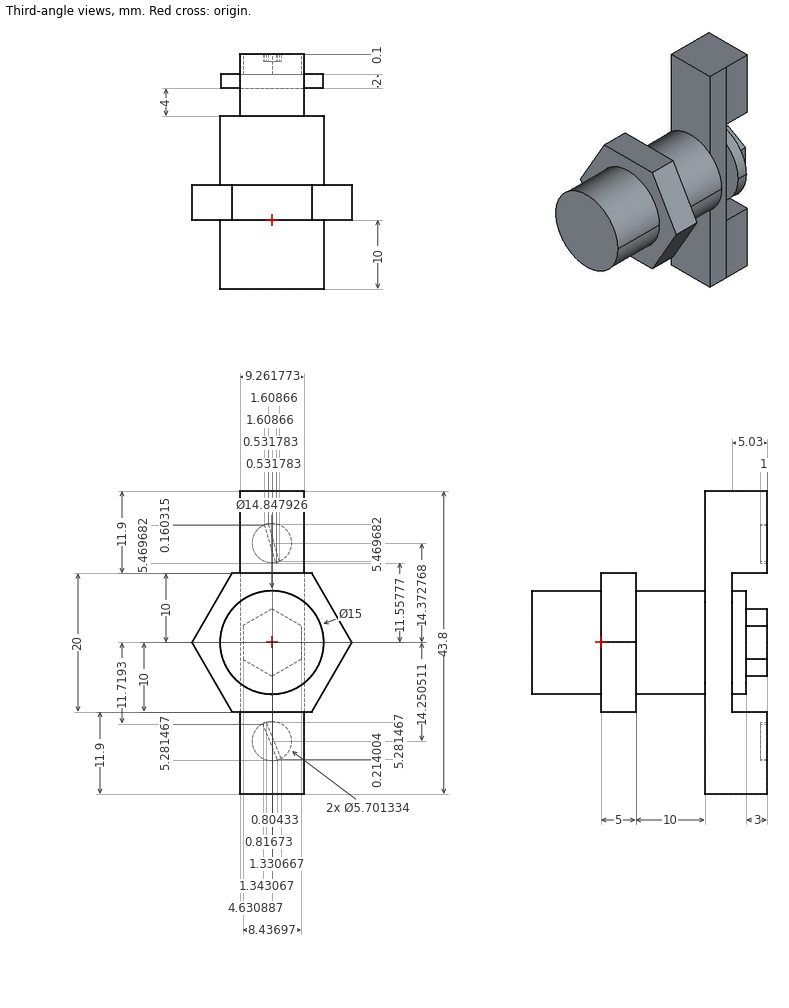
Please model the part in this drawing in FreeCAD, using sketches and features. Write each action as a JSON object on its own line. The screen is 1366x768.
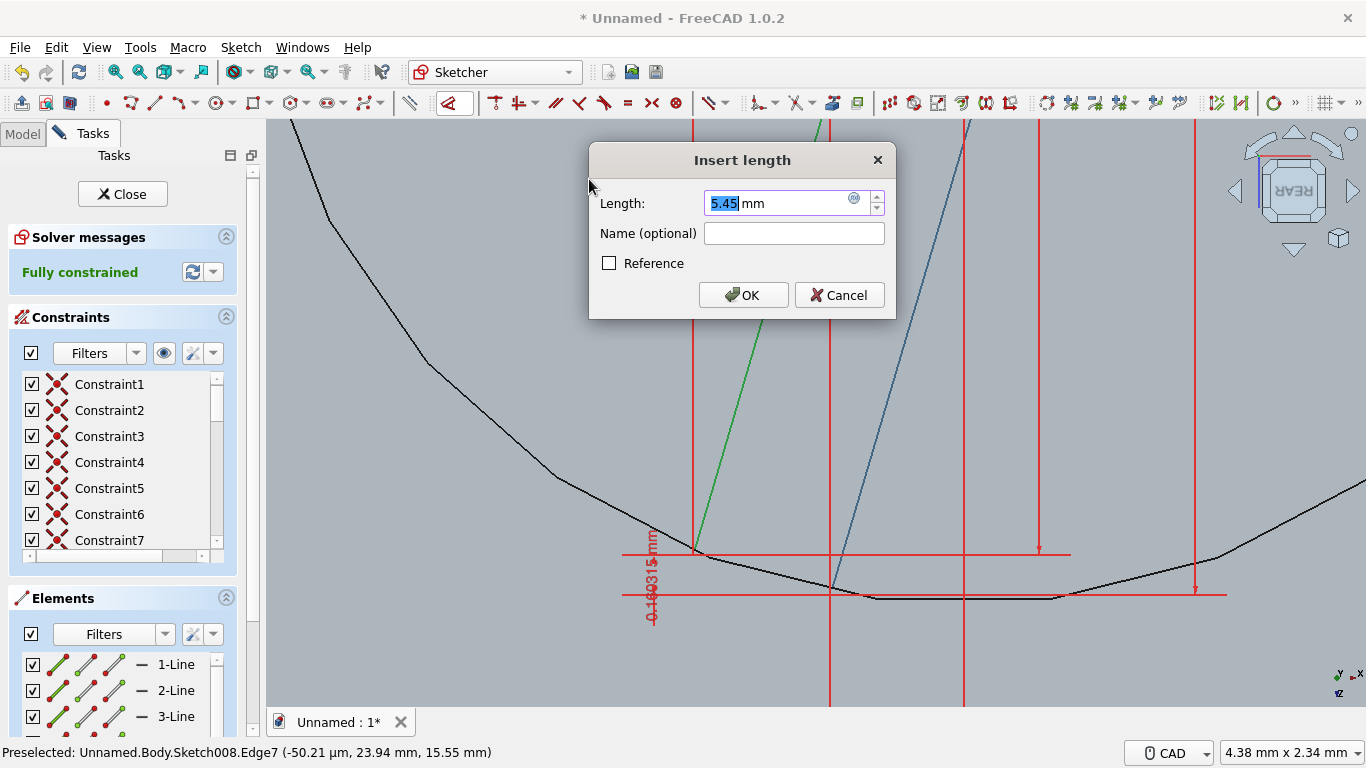
{"action": "type", "text": "5.469682"}
{"action": "key", "text": "Return"}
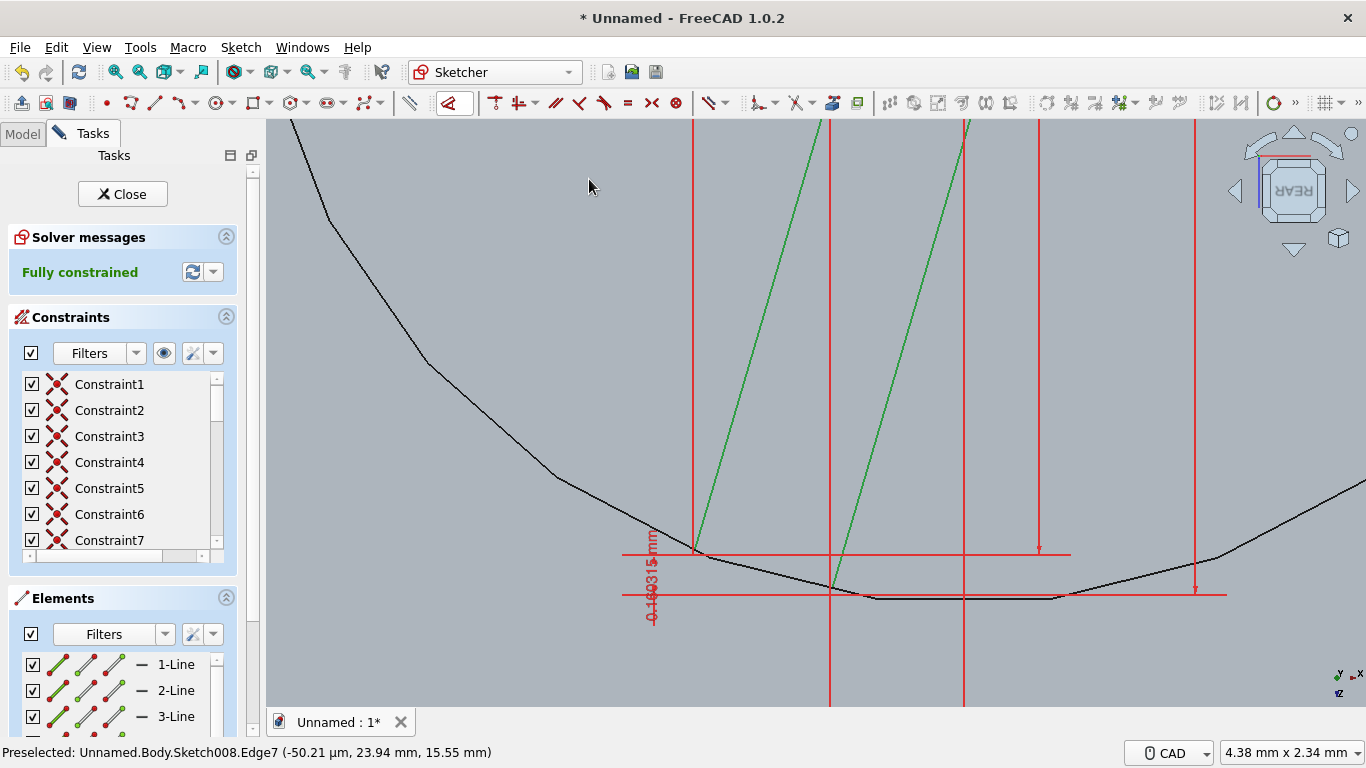
{"action": "left_click", "coordinate": [123, 194]}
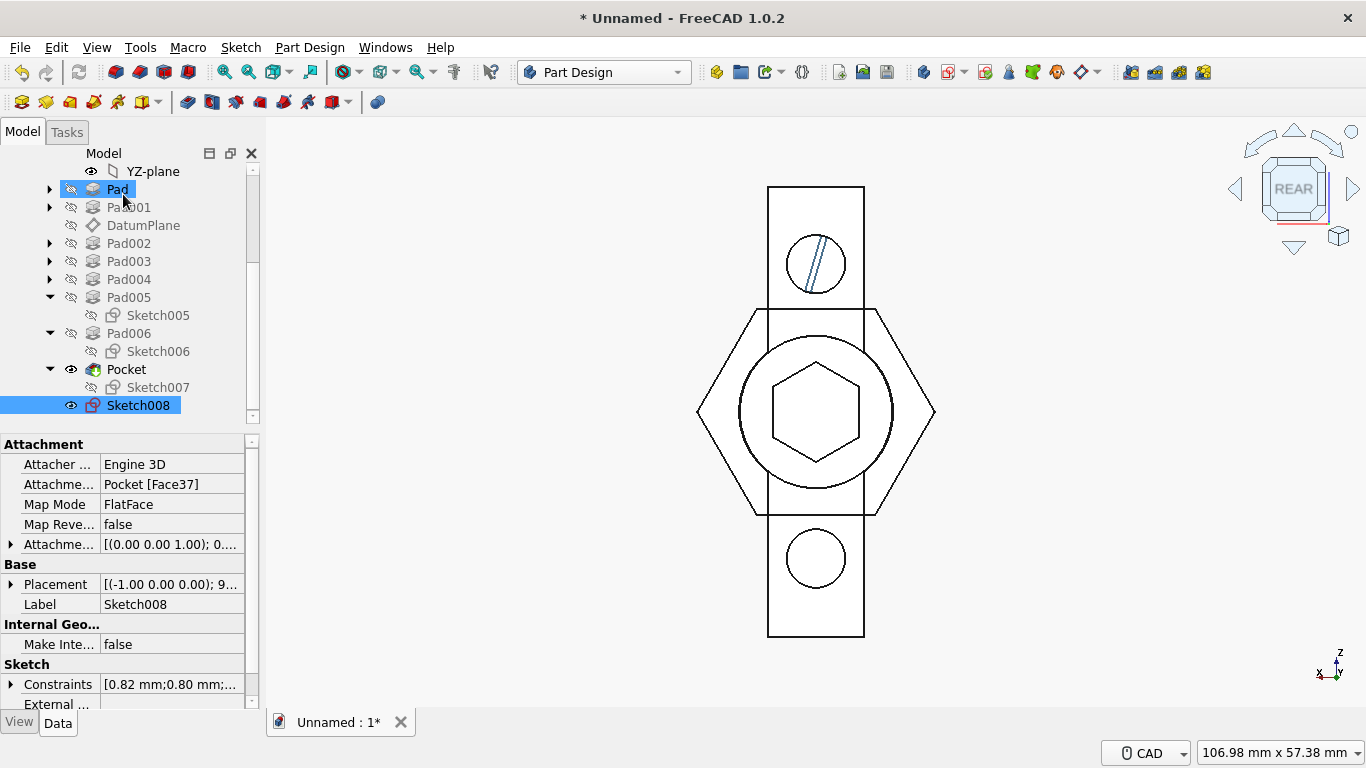
{"action": "left_click", "coordinate": [188, 102]}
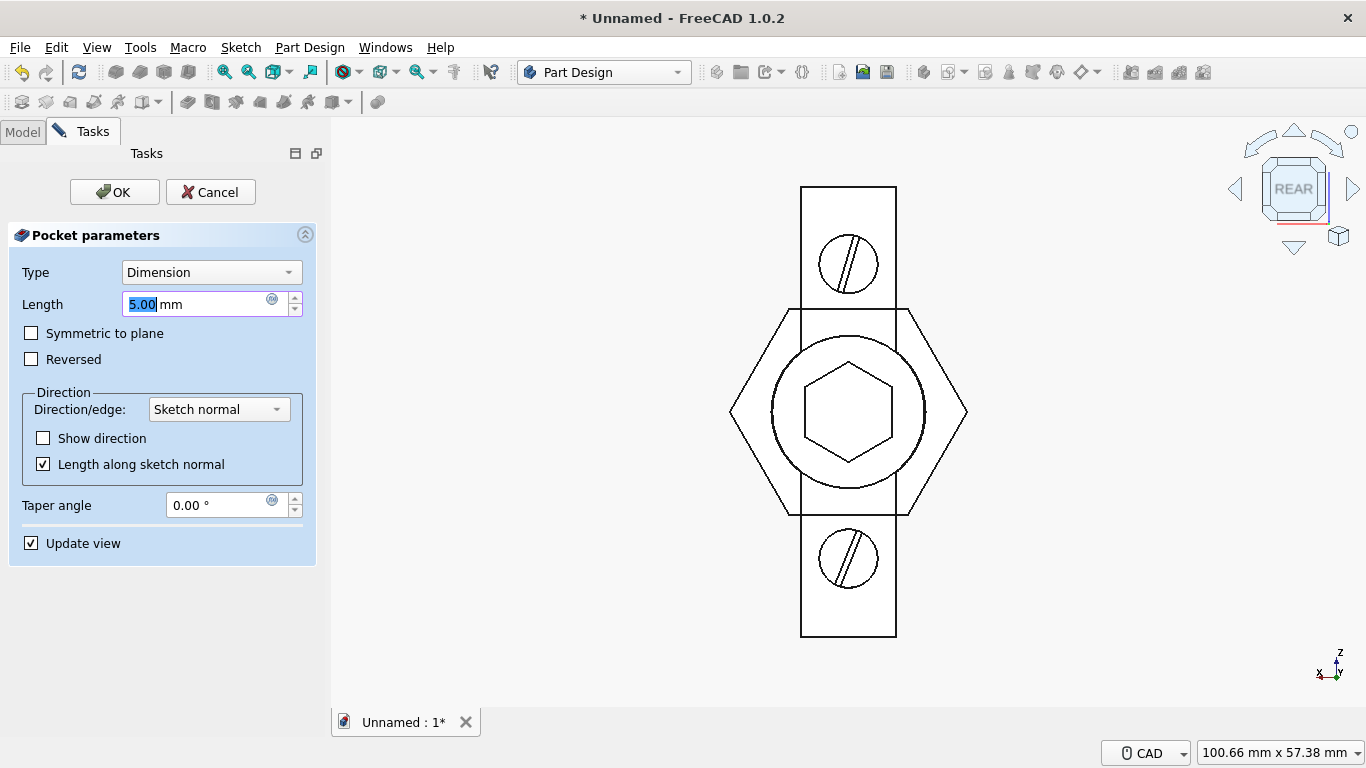
{"action": "type", "text": "1"}
{"action": "key", "text": "Tab"}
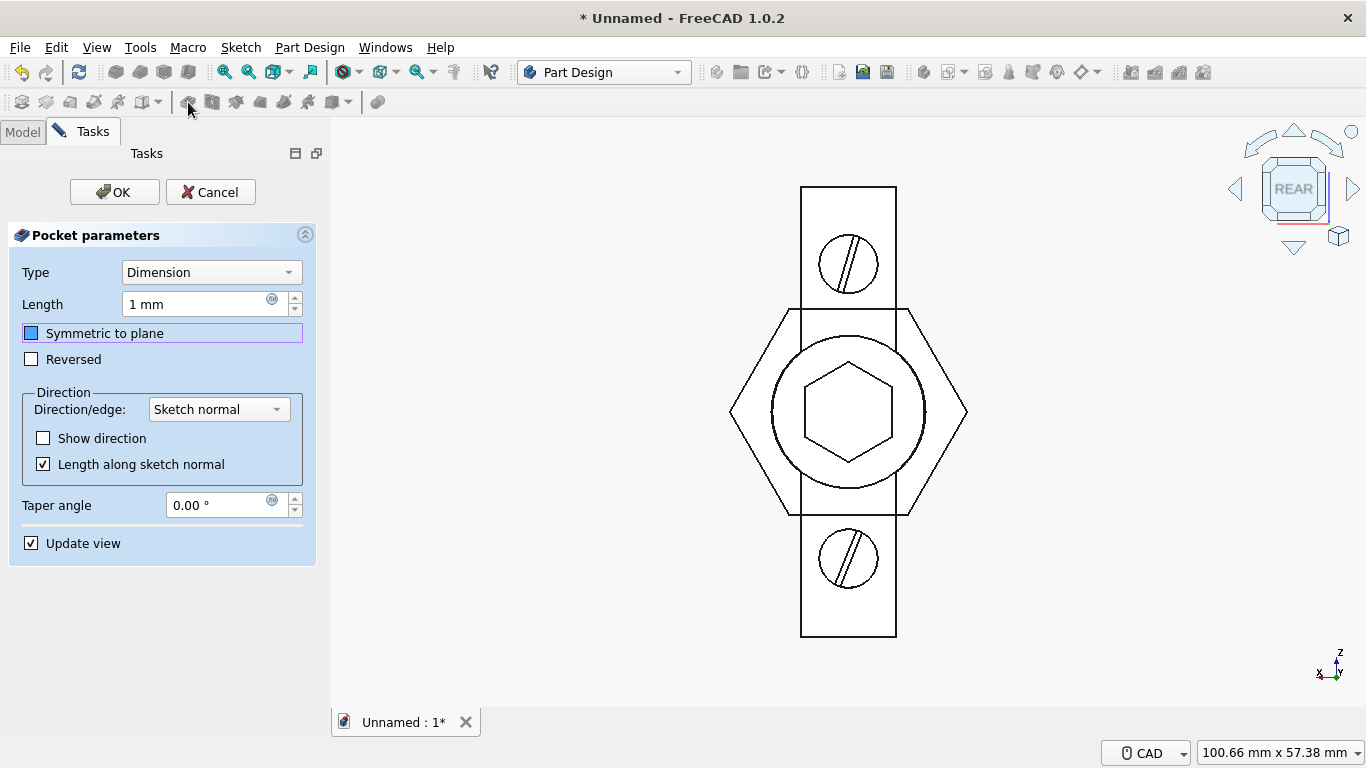
{"action": "left_click", "coordinate": [115, 192]}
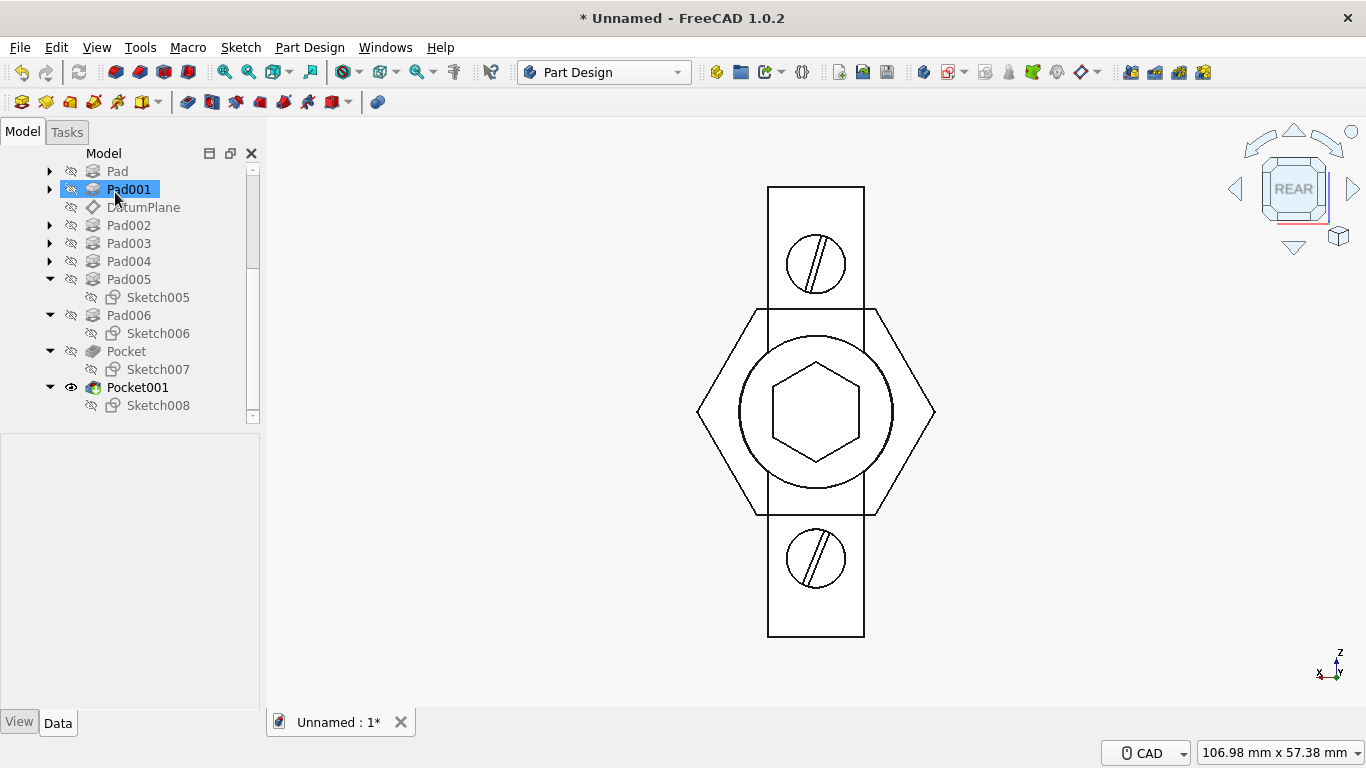
{"action": "key", "text": "0"}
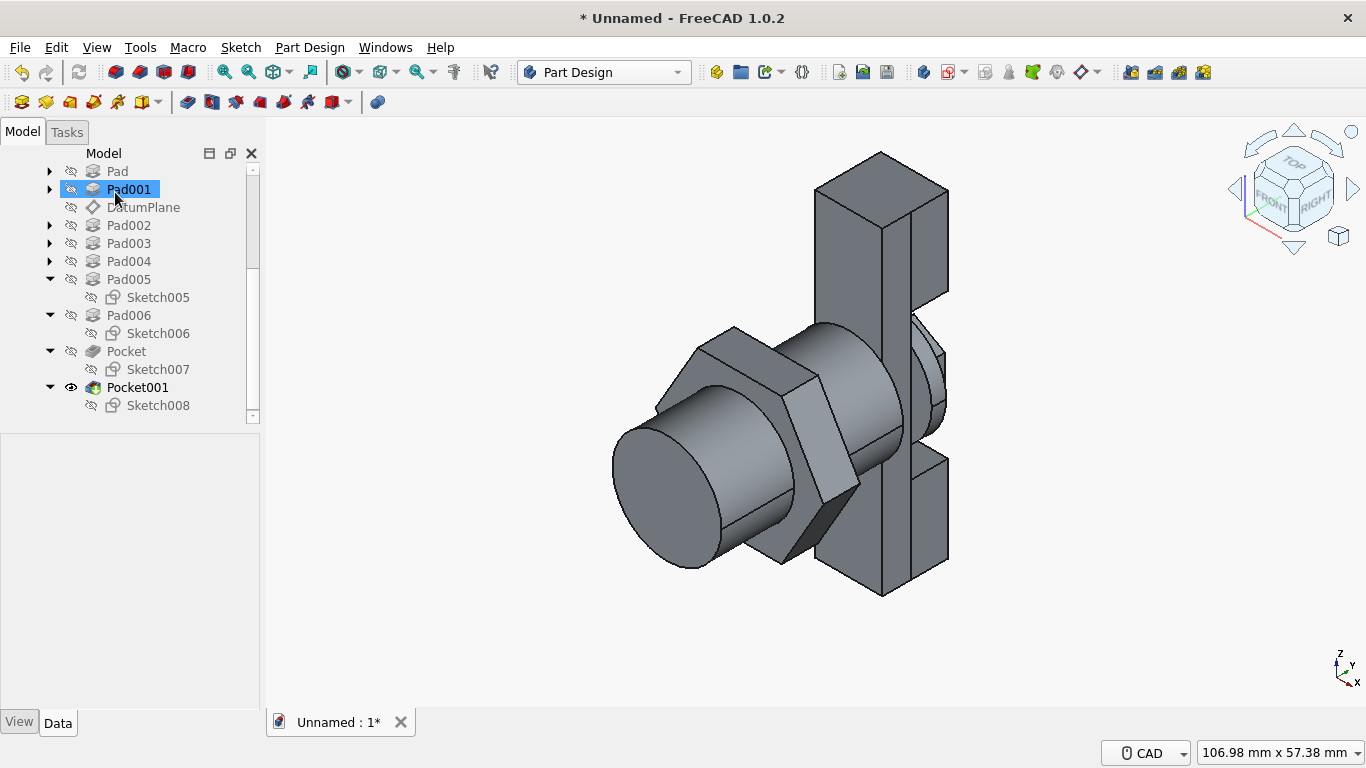
{"action": "left_click", "coordinate": [226, 72]}